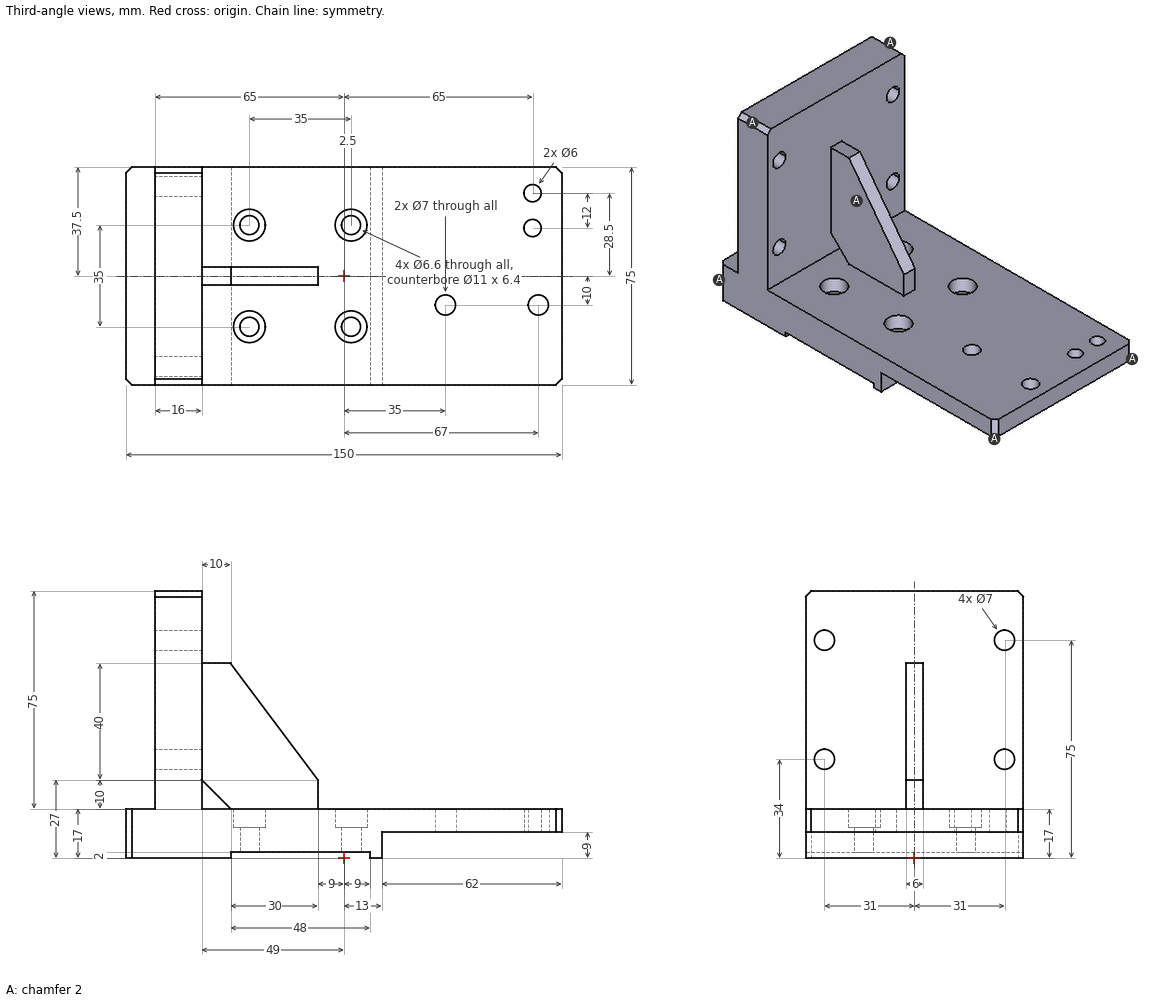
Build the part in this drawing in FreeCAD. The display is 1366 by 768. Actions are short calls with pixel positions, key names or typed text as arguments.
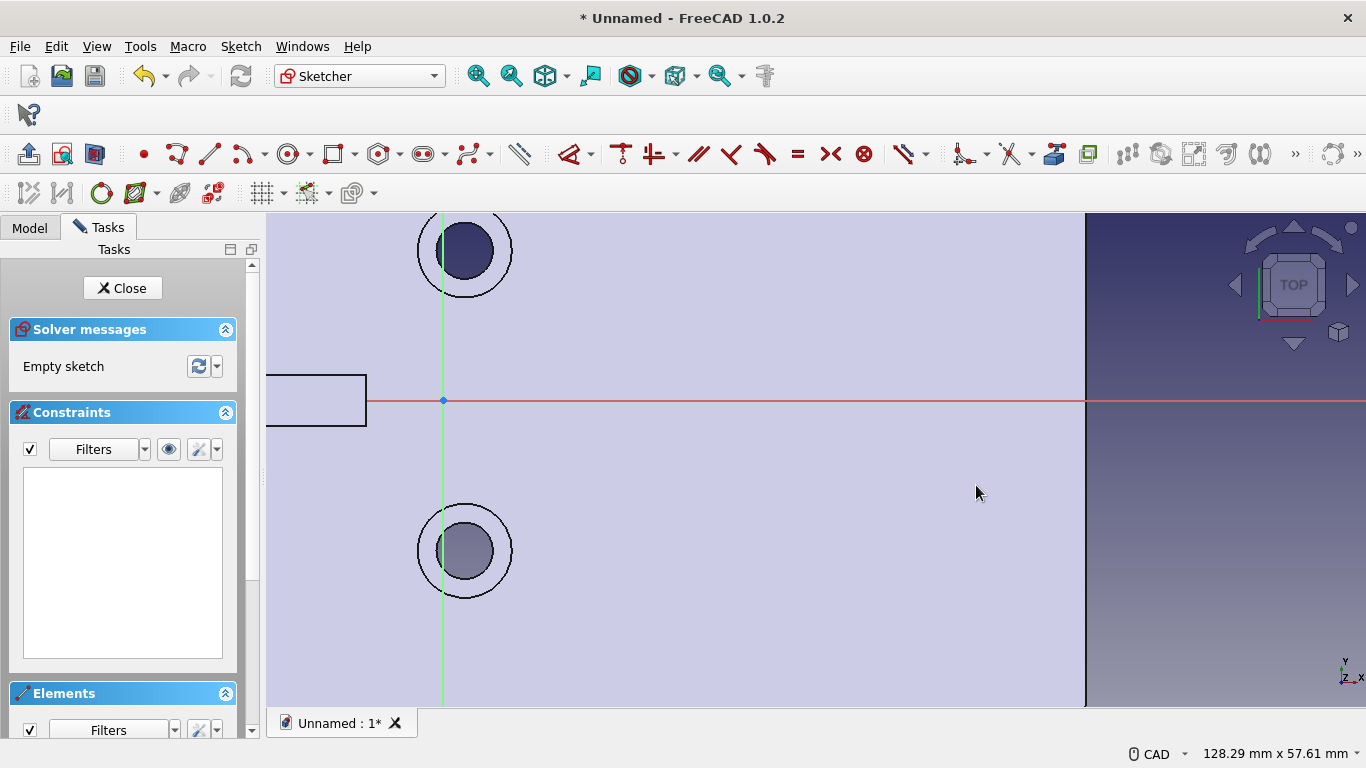
click(288, 154)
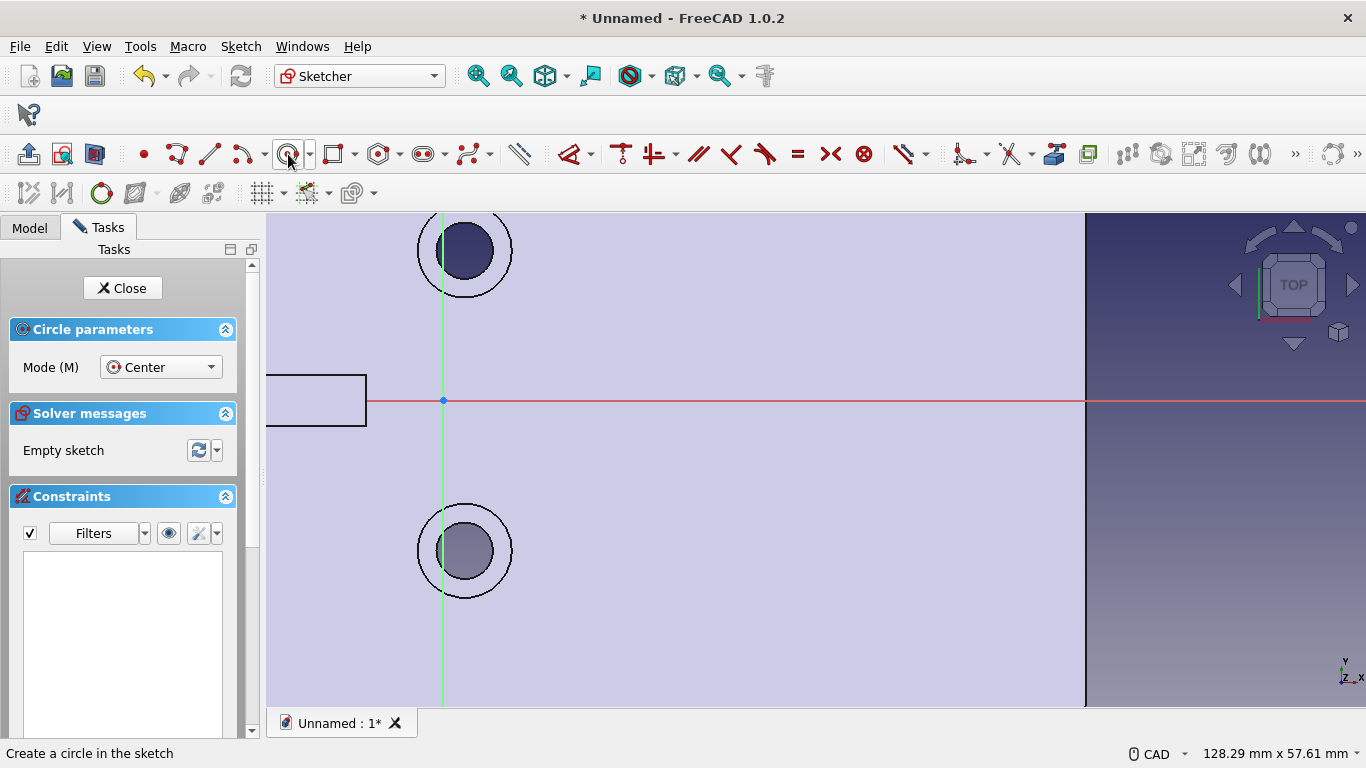
click(743, 486)
move(765, 465)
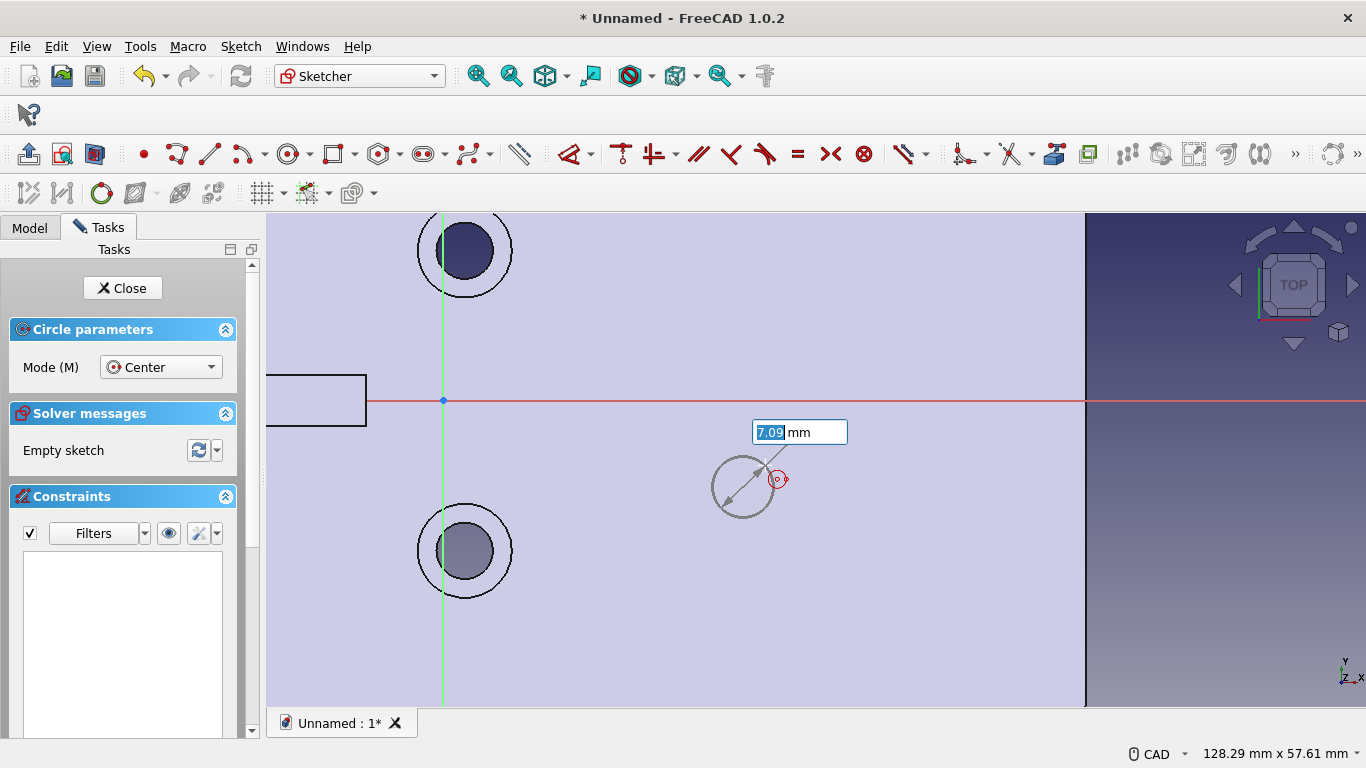
text(7)
key(Return)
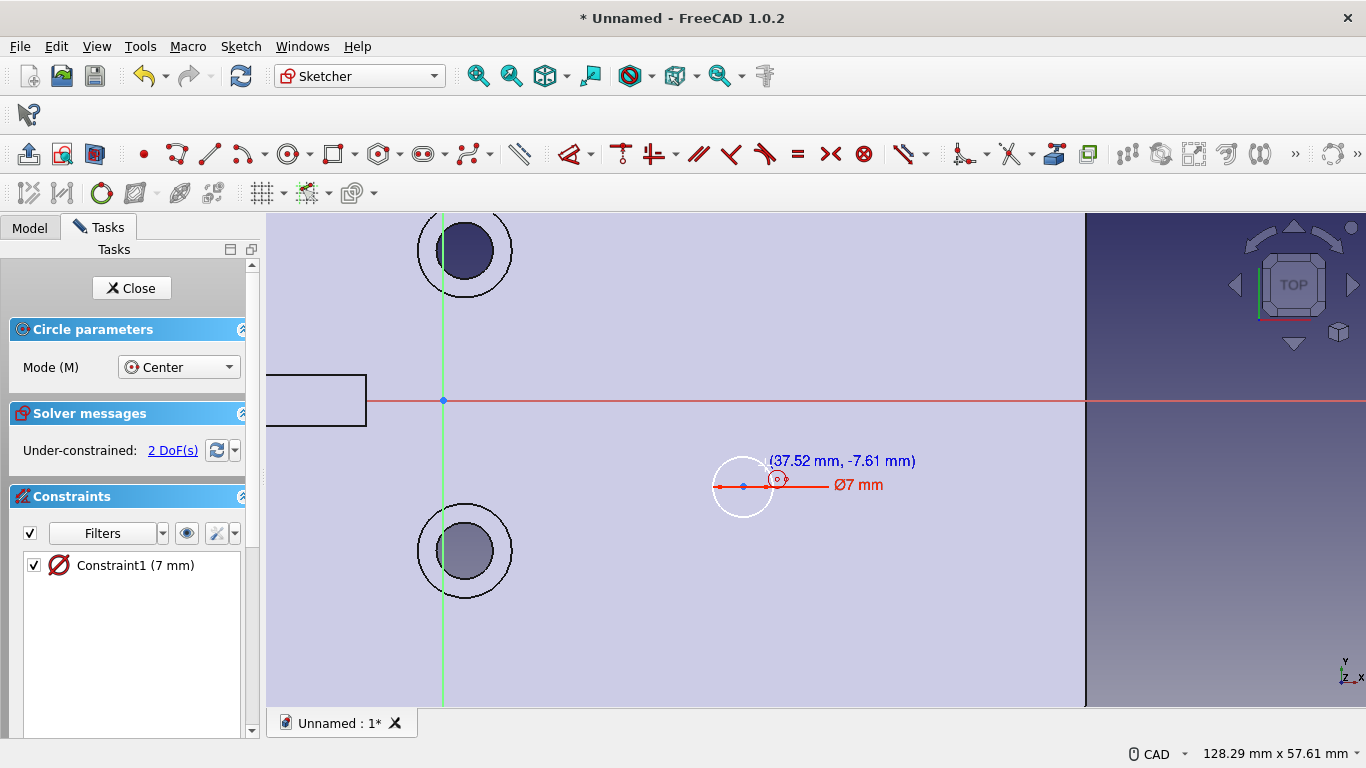
click(1018, 486)
move(1039, 465)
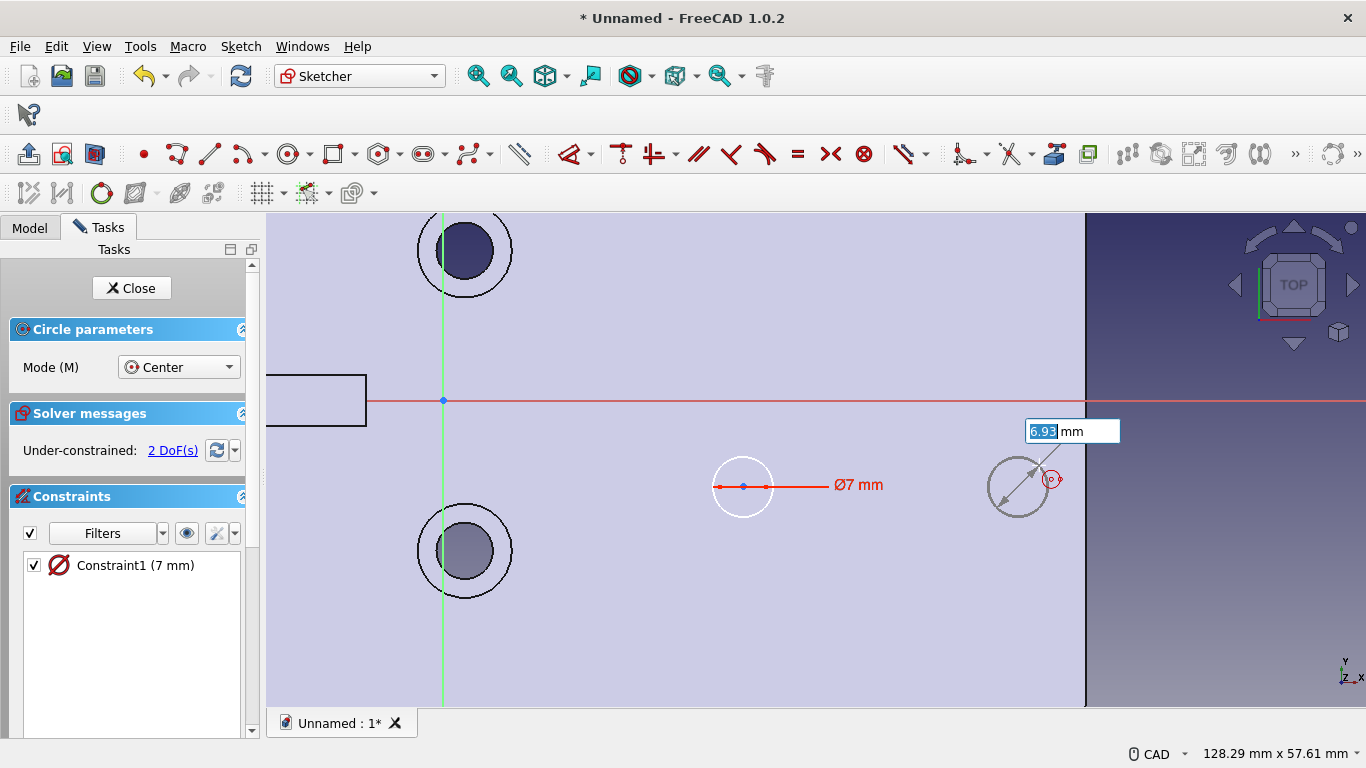
text(7)
key(Return)
key(Escape)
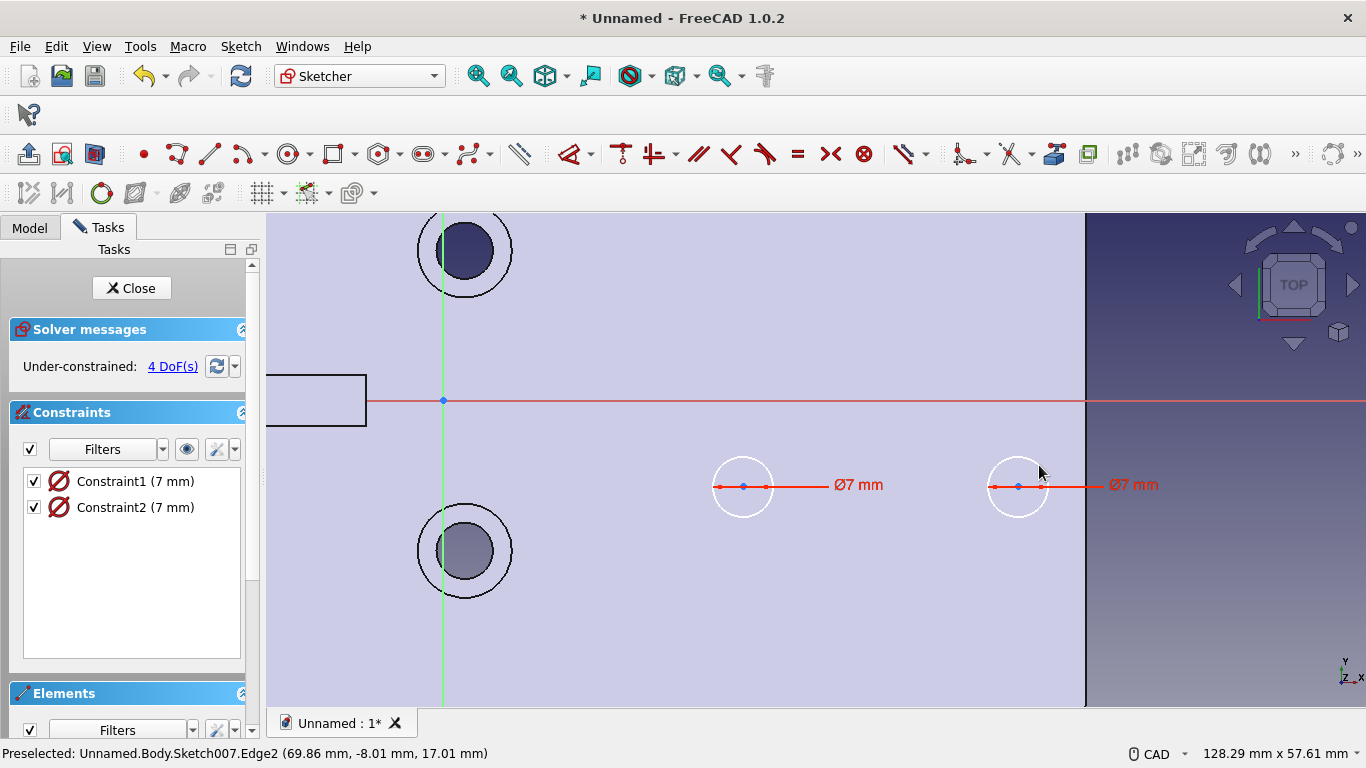
click(568, 154)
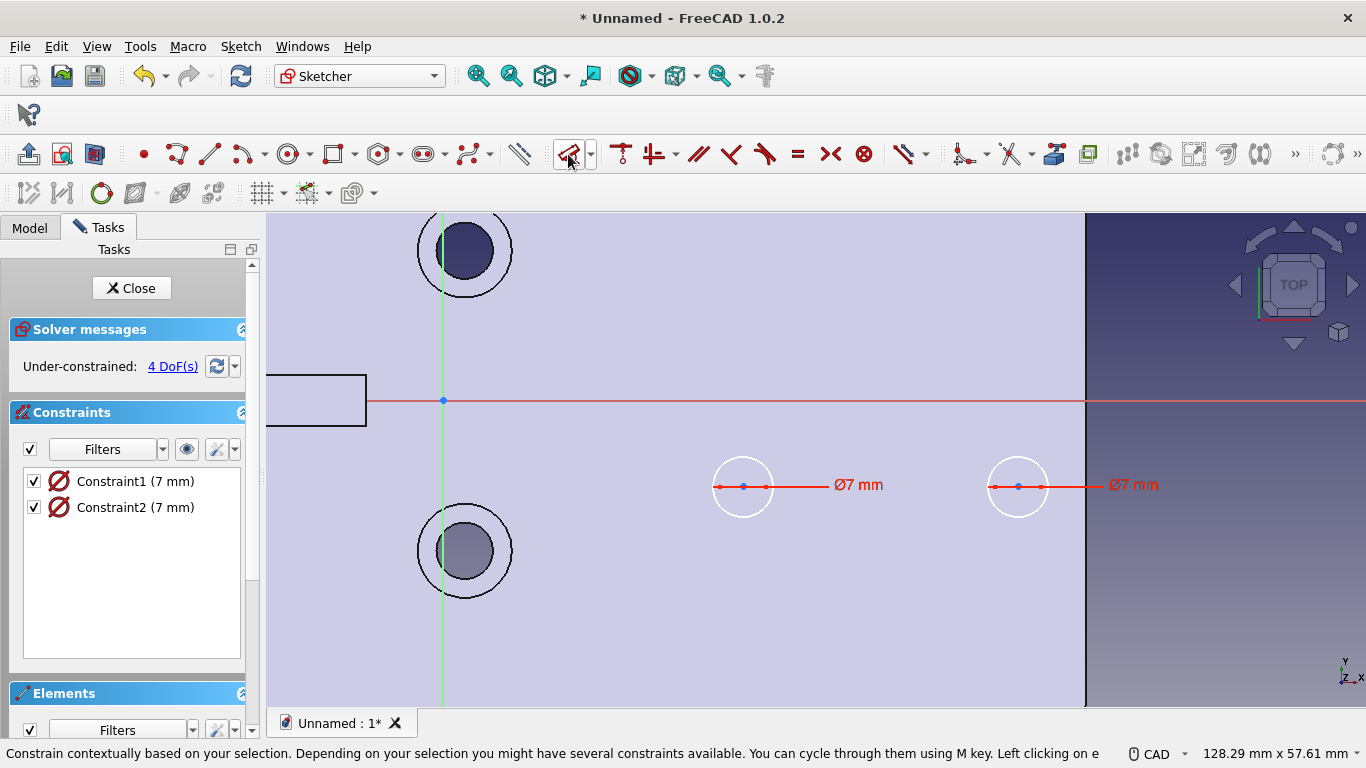
click(743, 487)
click(593, 367)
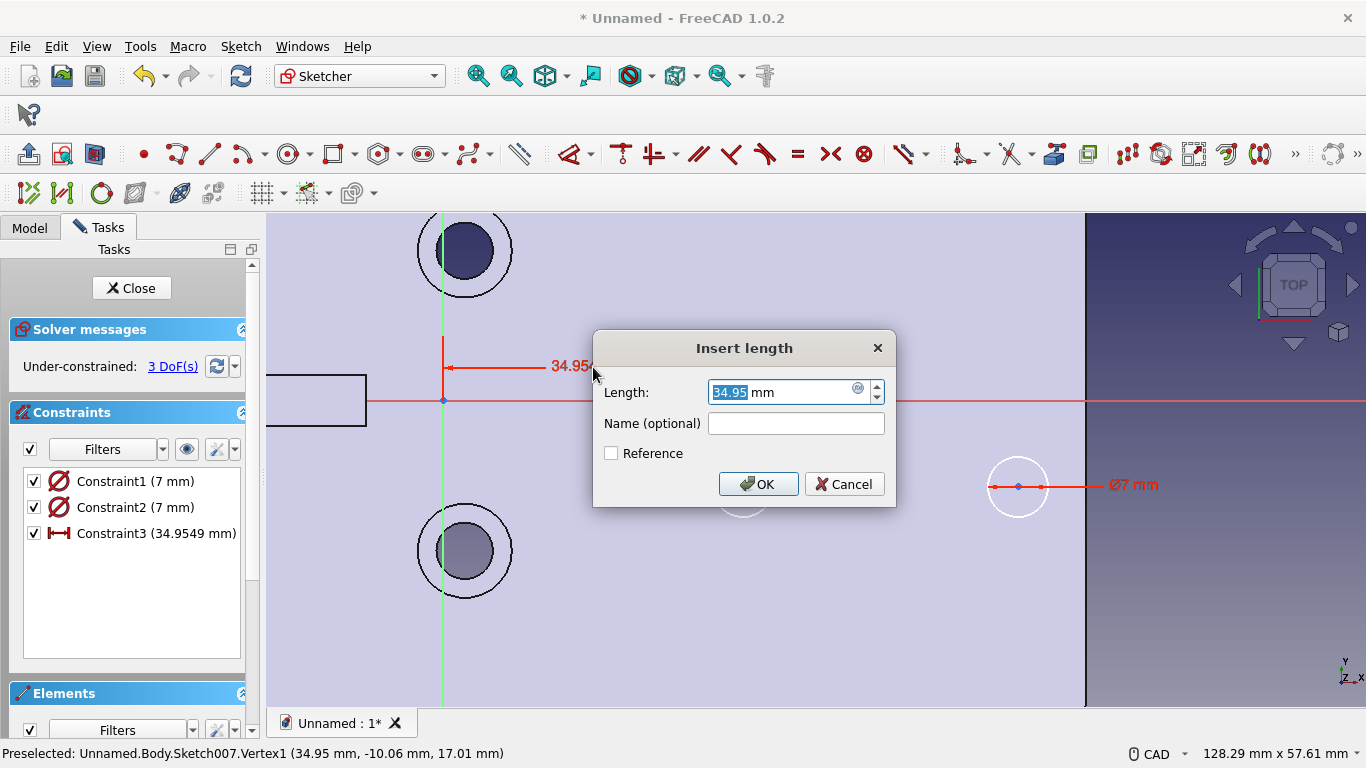
text(35)
key(Return)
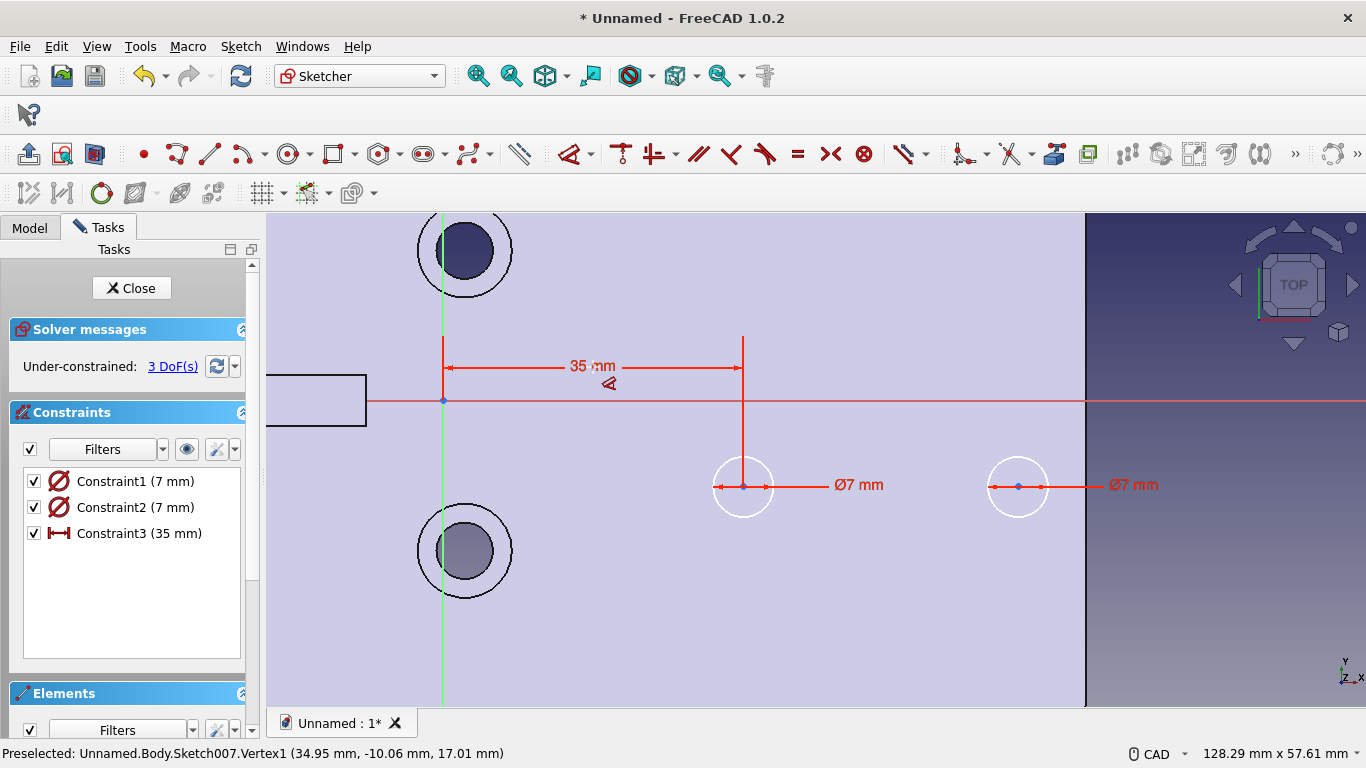
click(743, 487)
click(409, 444)